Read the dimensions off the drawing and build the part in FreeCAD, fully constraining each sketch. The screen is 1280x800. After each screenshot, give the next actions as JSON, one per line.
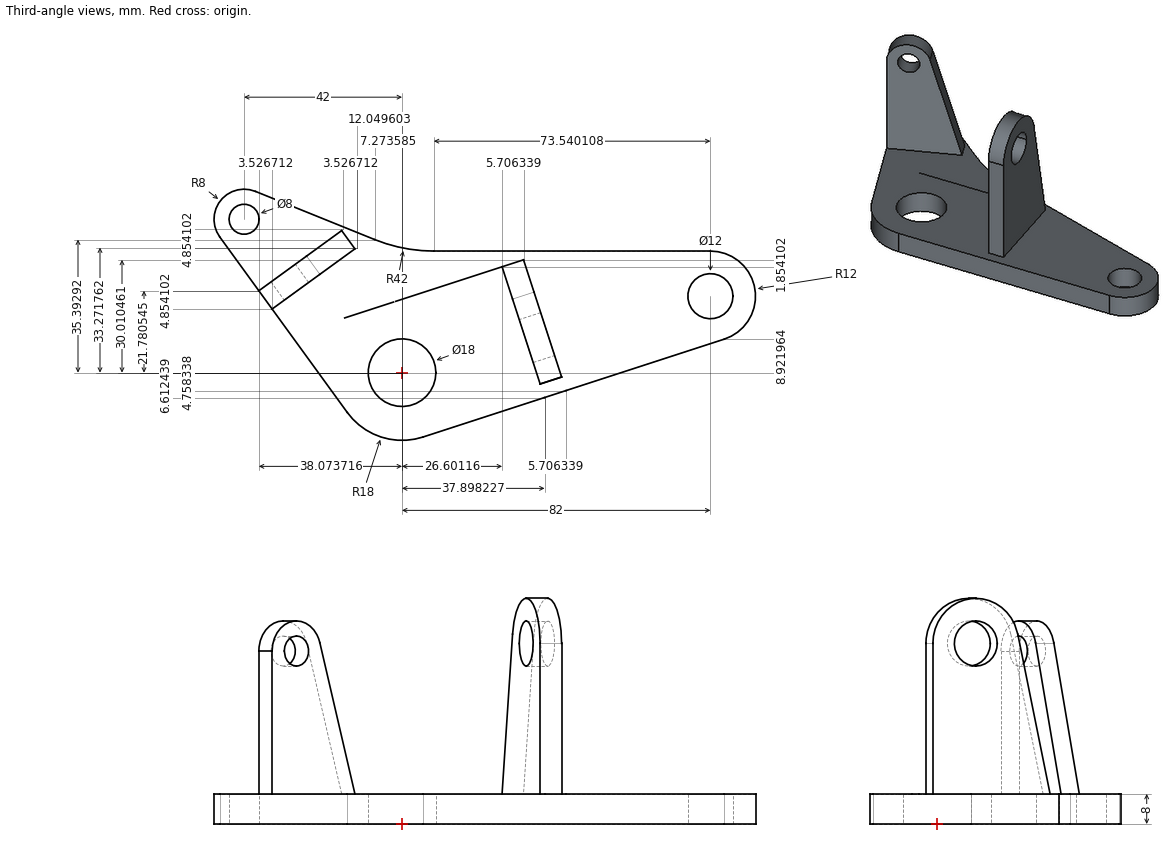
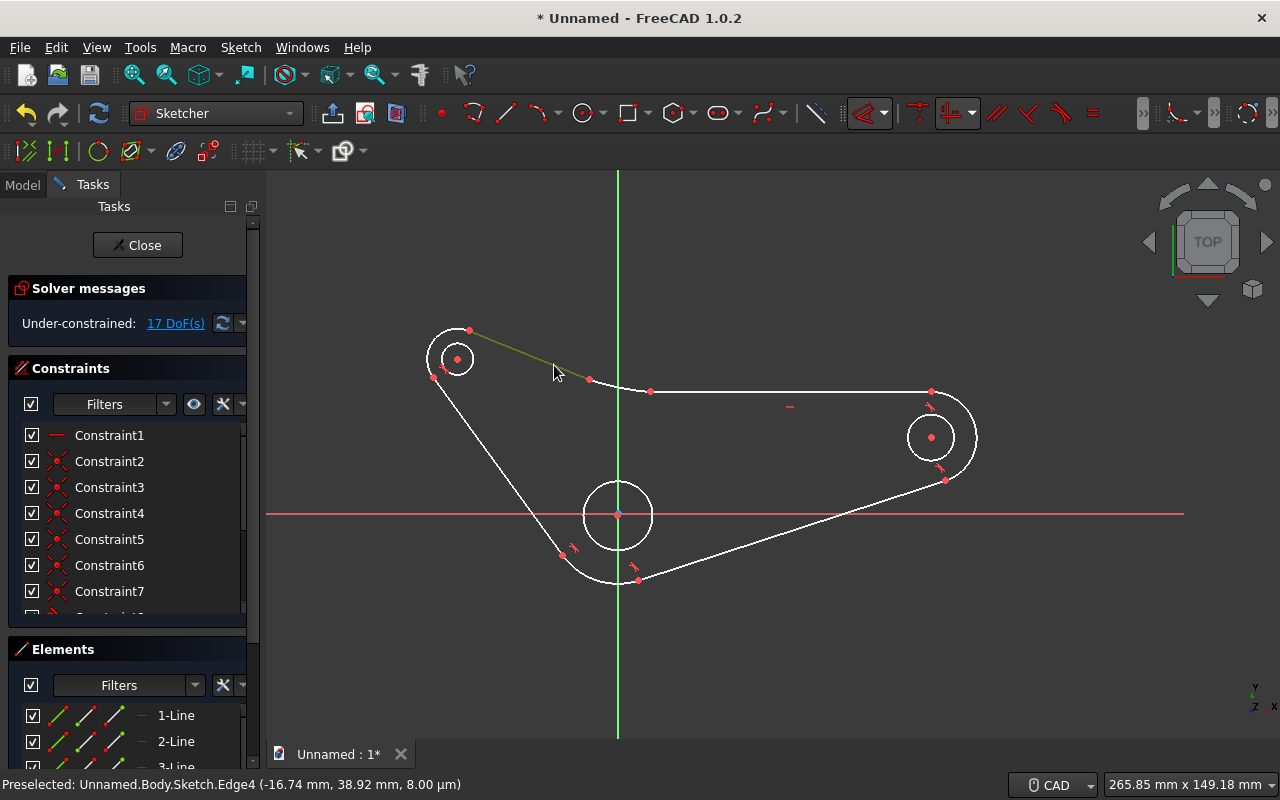
{"action": "scroll", "coordinate": [608, 385], "scroll_direction": "up", "scroll_amount": 2}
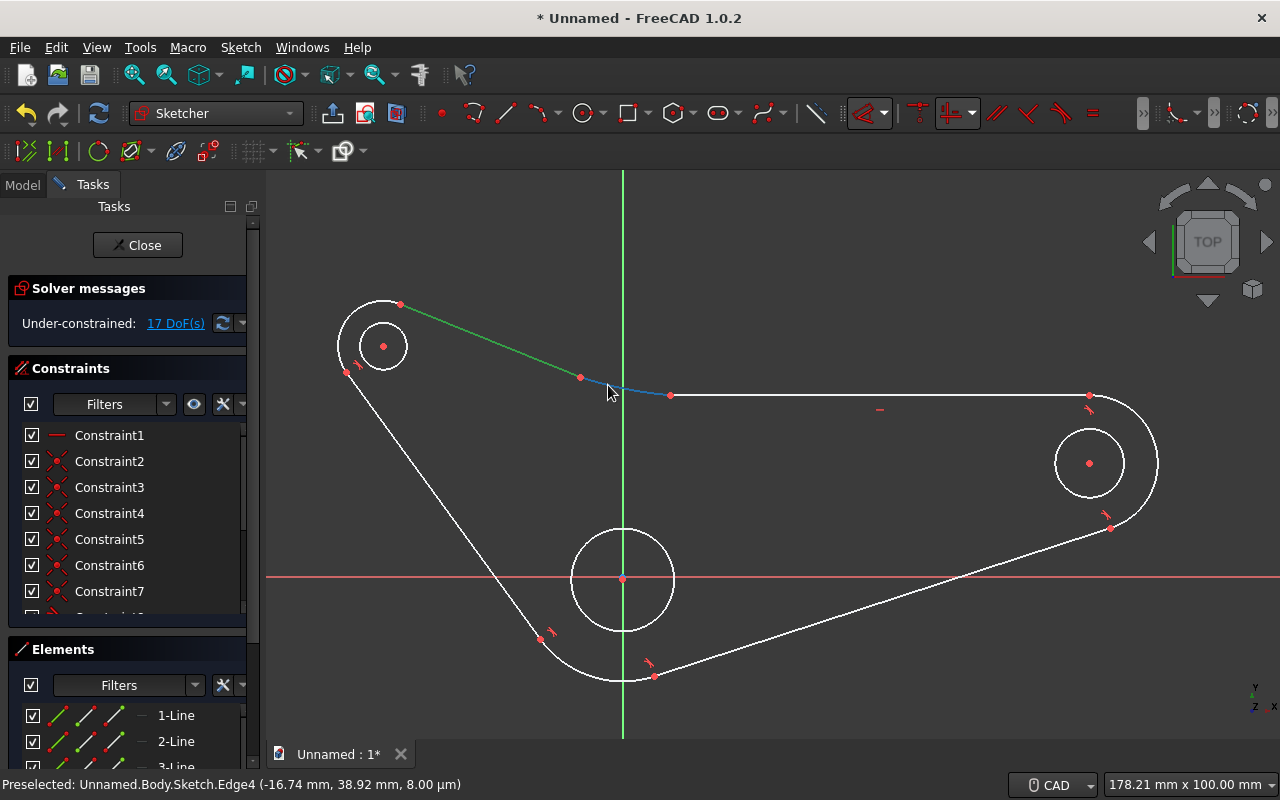
{"action": "left_click", "coordinate": [607, 385]}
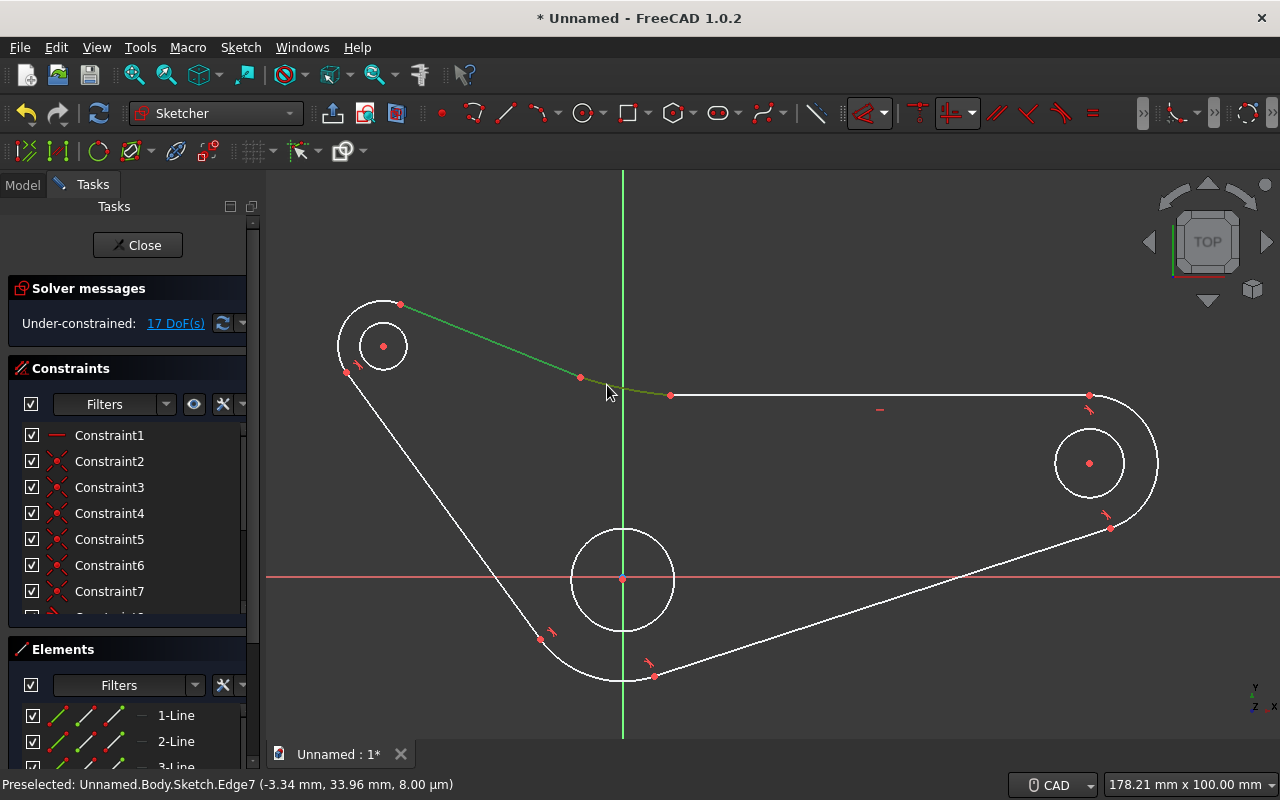
{"action": "key", "text": "t"}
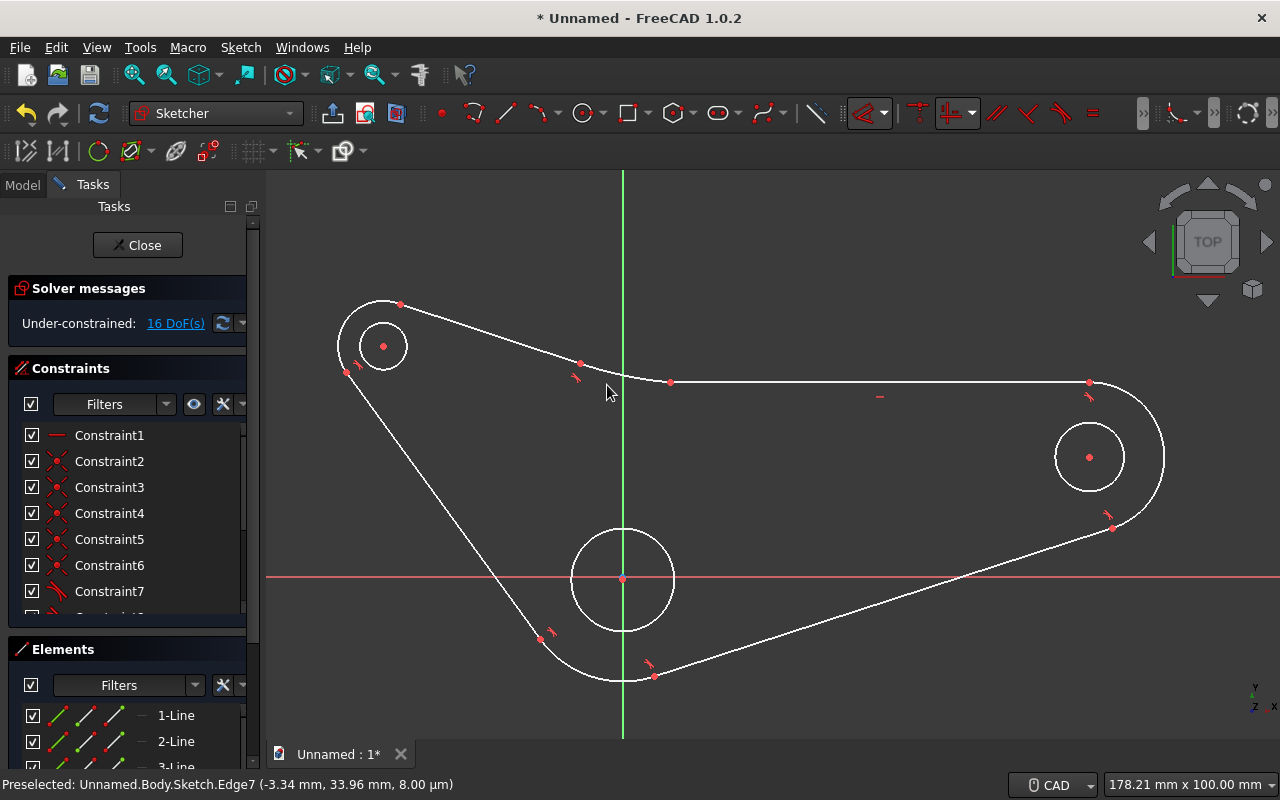
{"action": "left_click", "coordinate": [527, 346]}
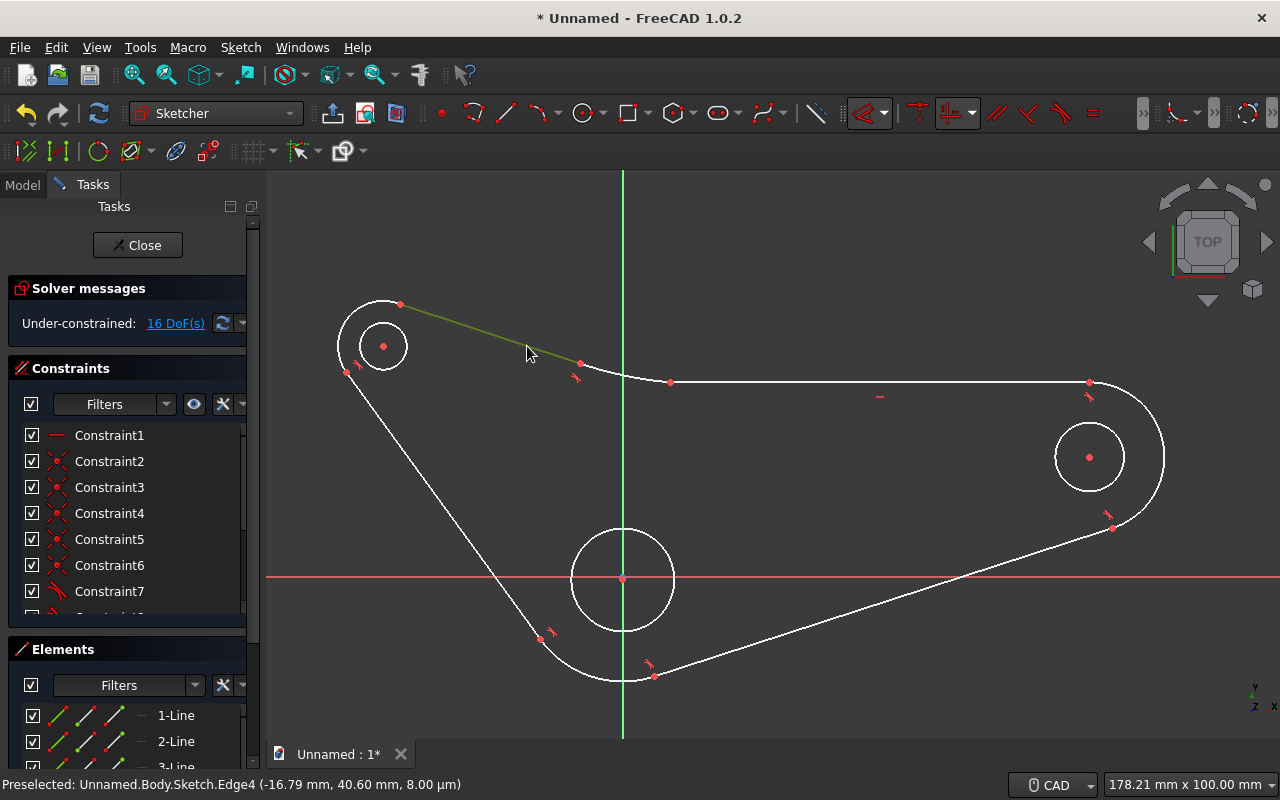
{"action": "left_click", "coordinate": [366, 304]}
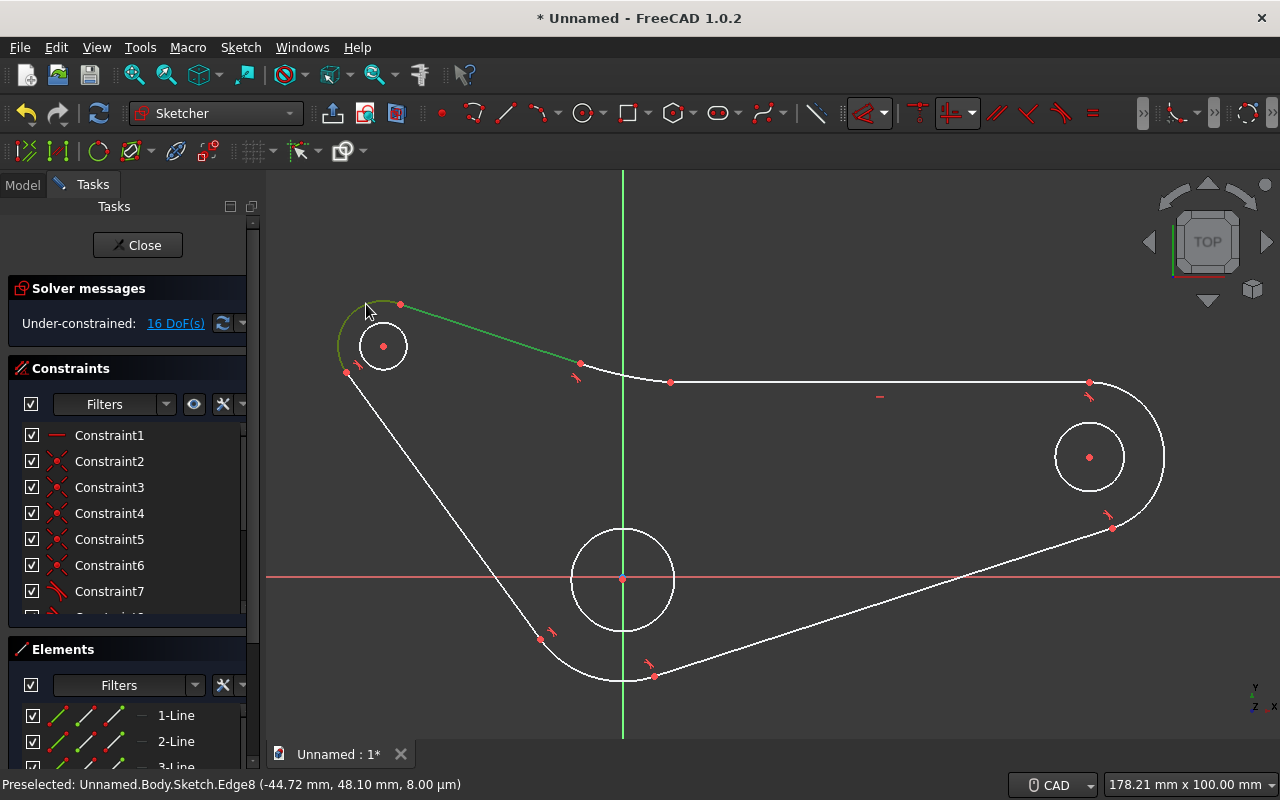
{"action": "key", "text": "t"}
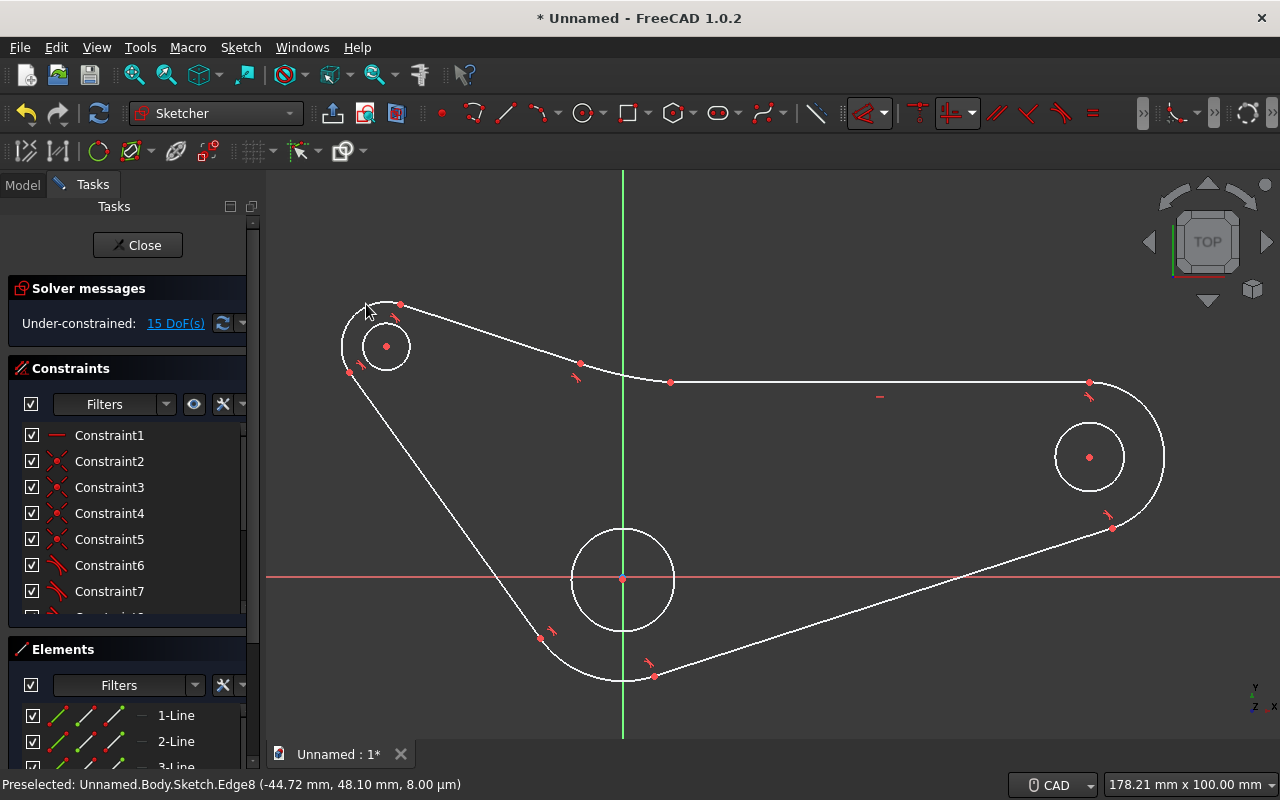
{"action": "scroll", "coordinate": [623, 579], "scroll_direction": "up", "scroll_amount": 3}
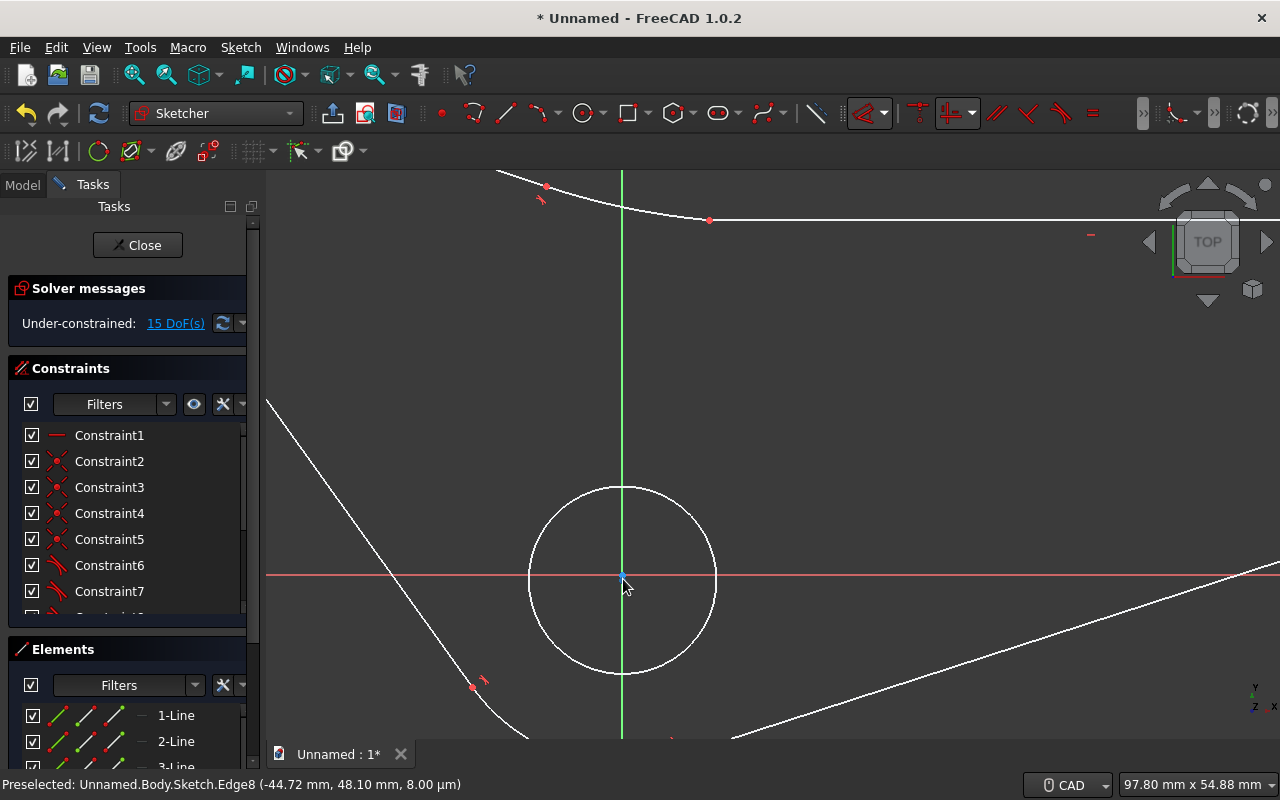
{"action": "left_click_drag", "start_coordinate": [612, 565], "coordinate": [633, 590]}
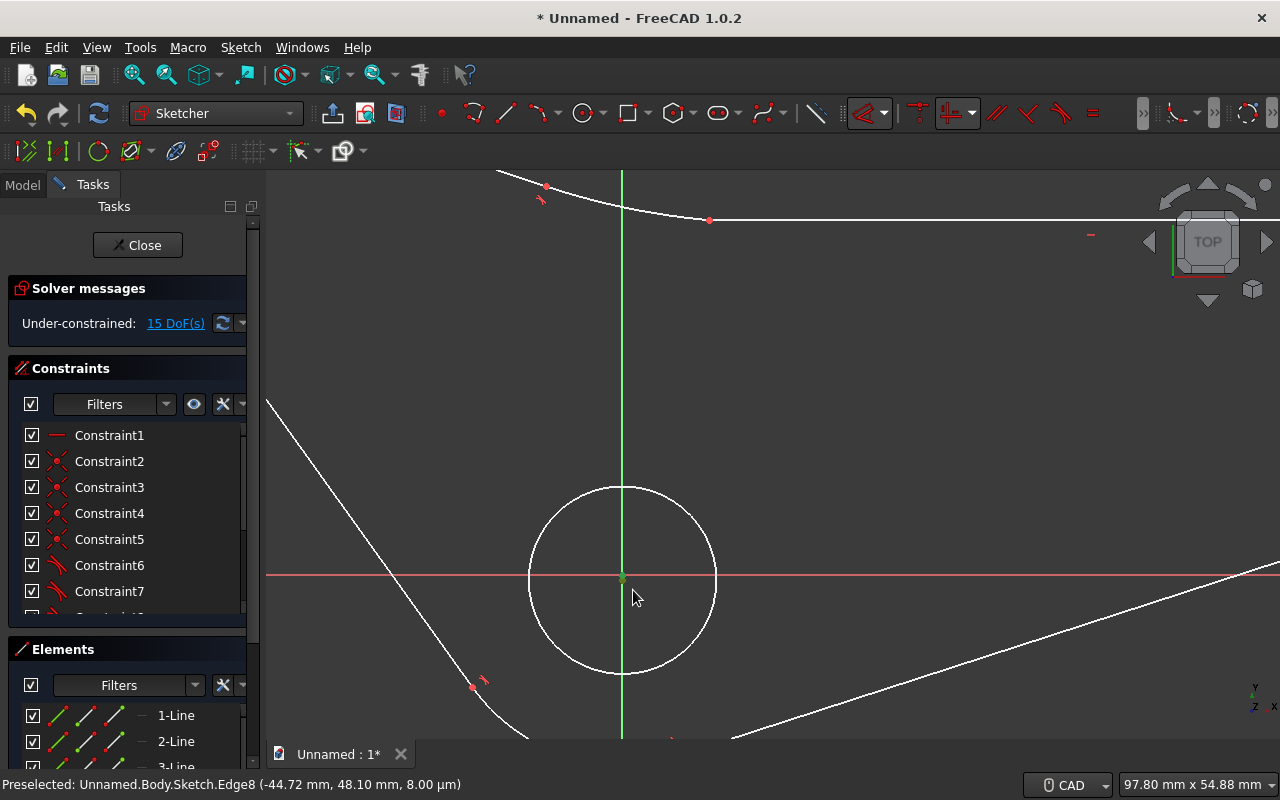
{"action": "key", "text": "c"}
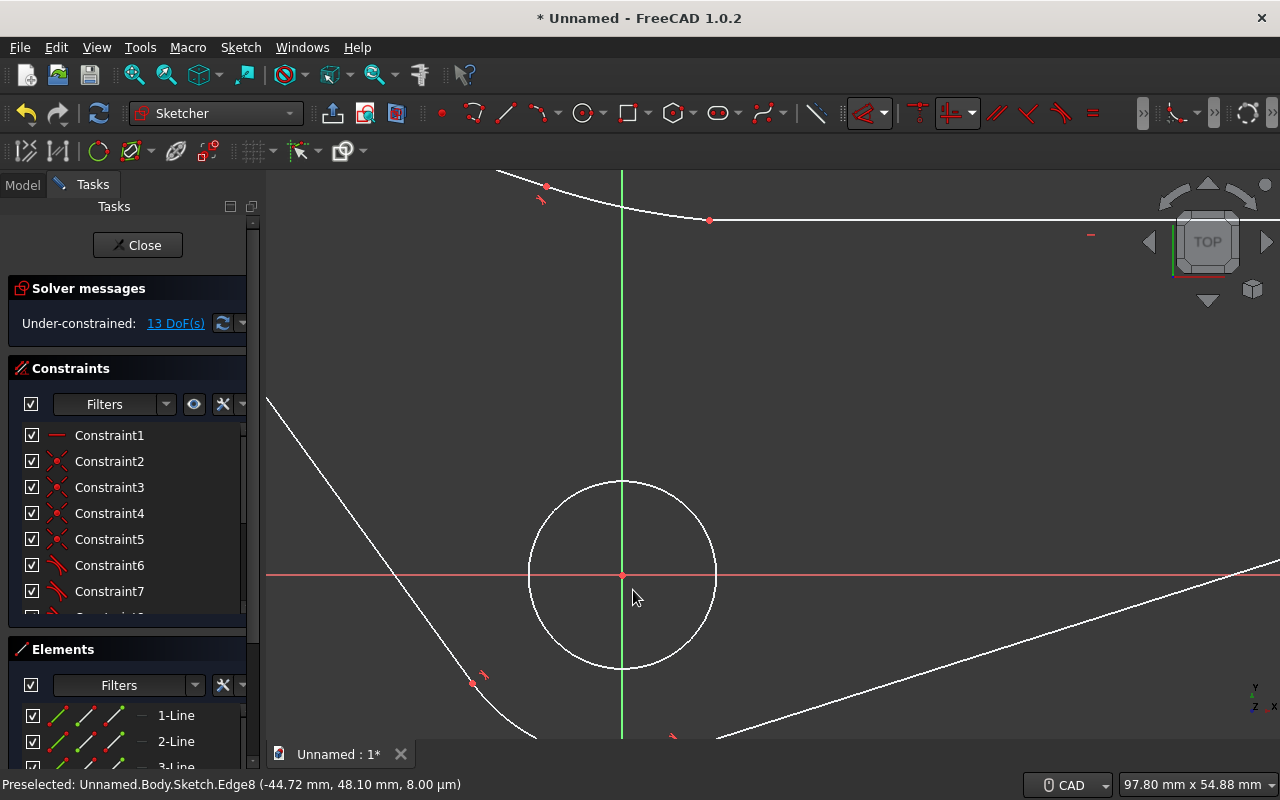
{"action": "scroll", "coordinate": [615, 478], "scroll_direction": "down", "scroll_amount": 5}